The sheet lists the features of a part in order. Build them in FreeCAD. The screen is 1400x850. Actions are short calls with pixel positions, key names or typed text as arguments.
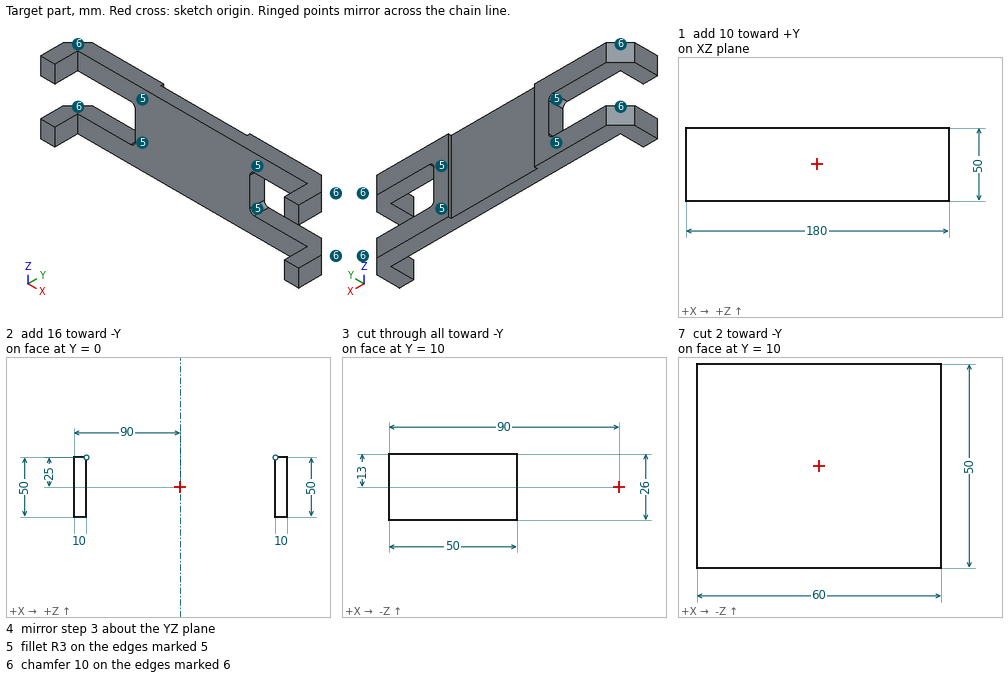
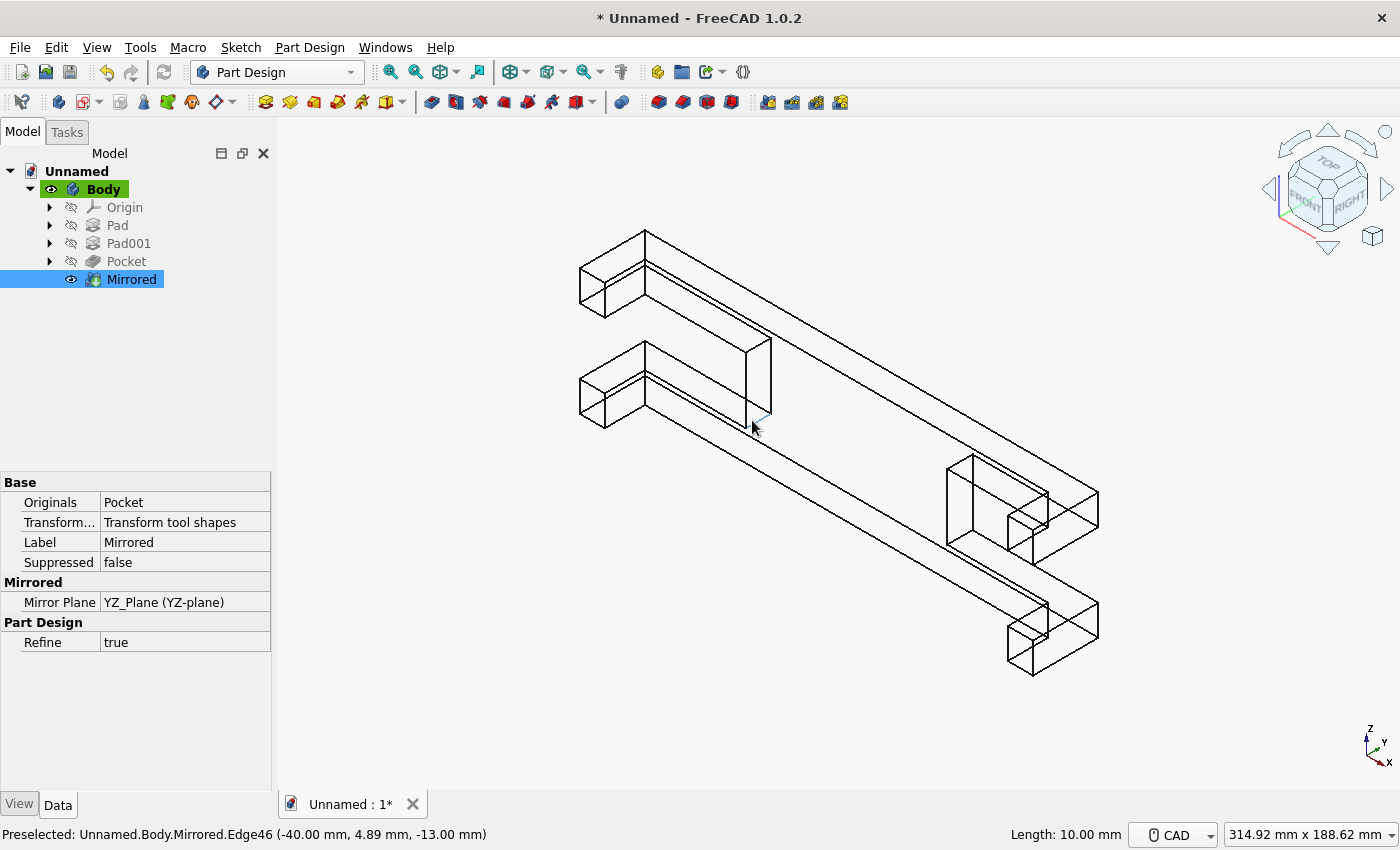
click(758, 344, ctrl)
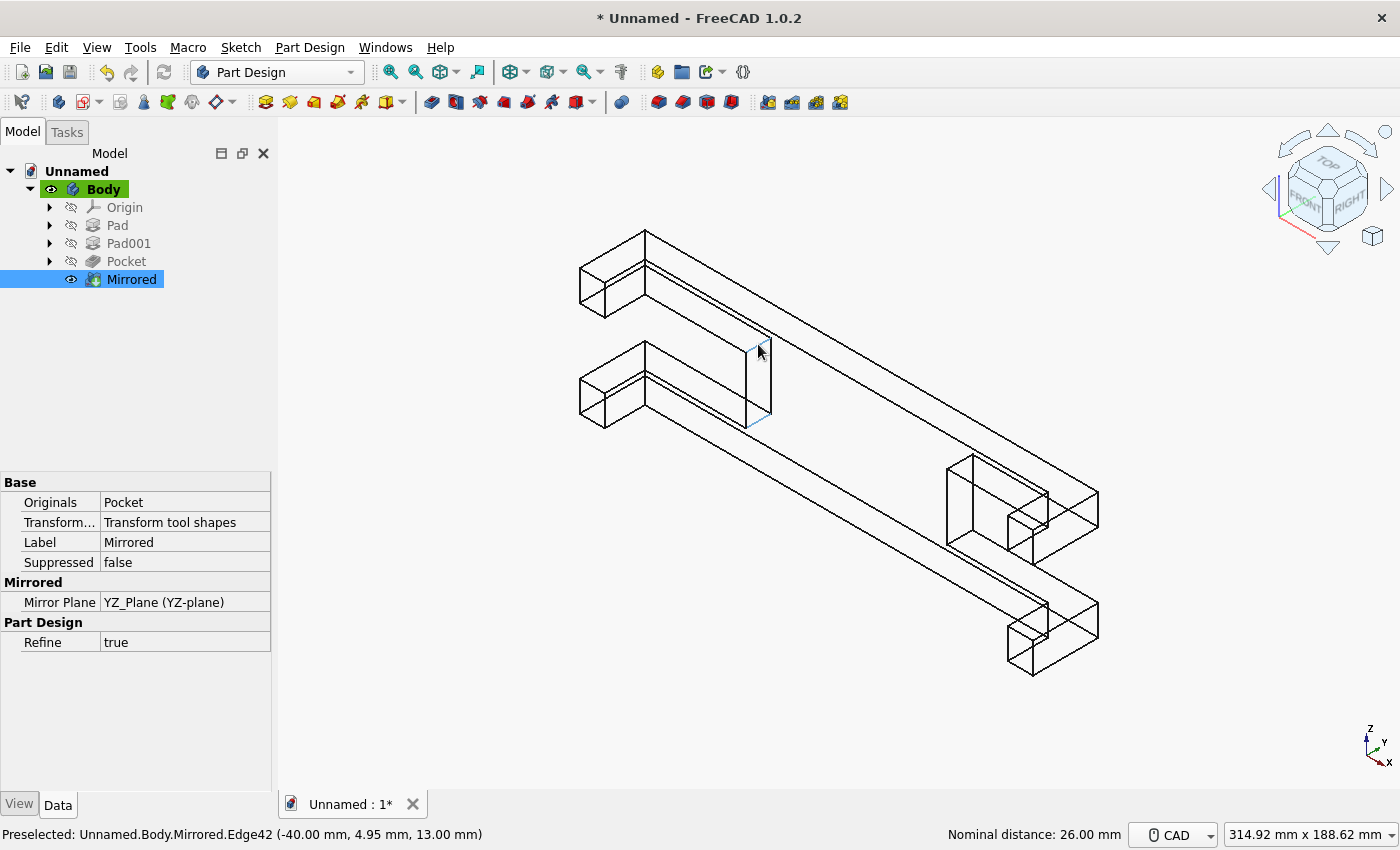
click(960, 461, ctrl)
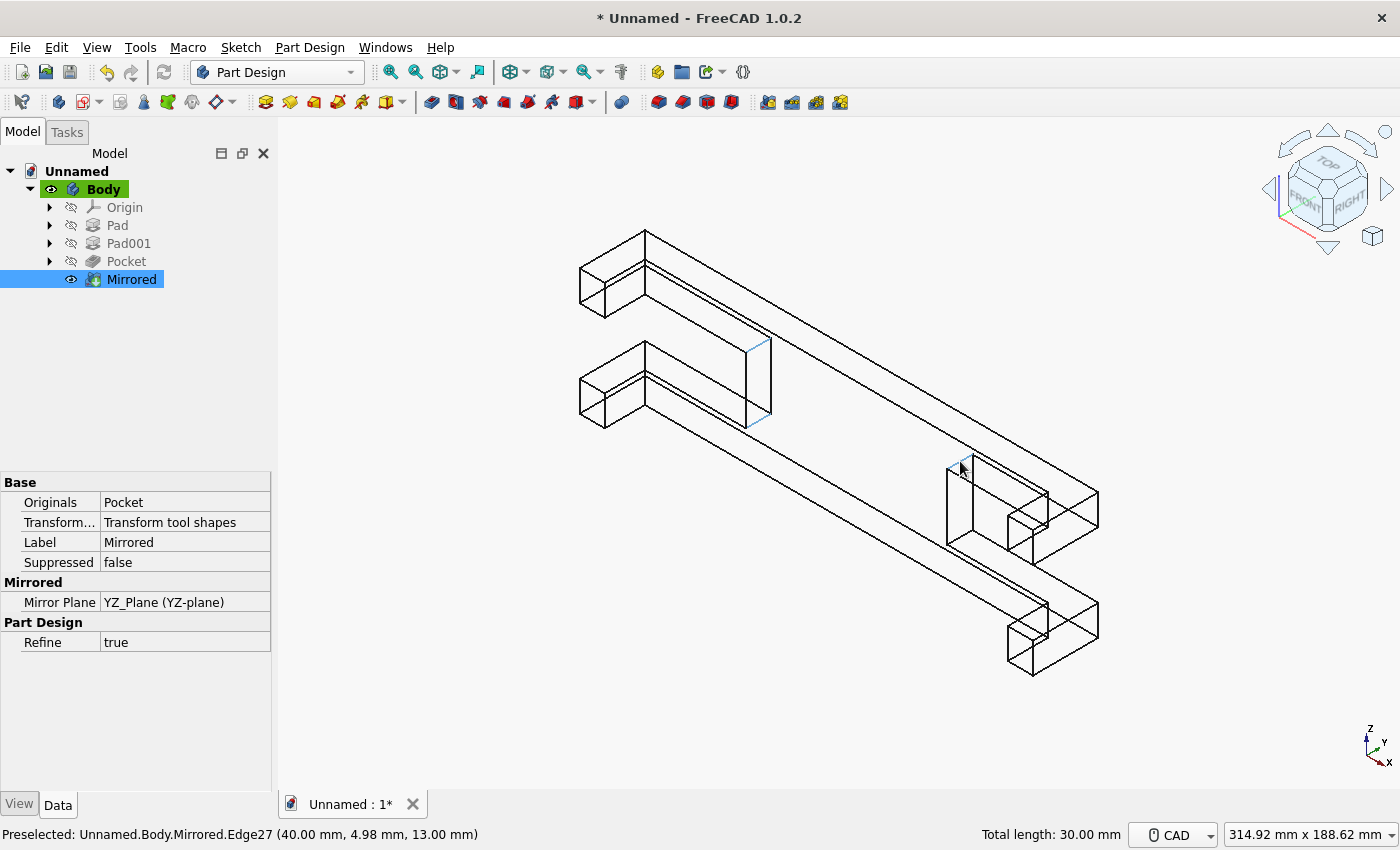
click(960, 536, ctrl)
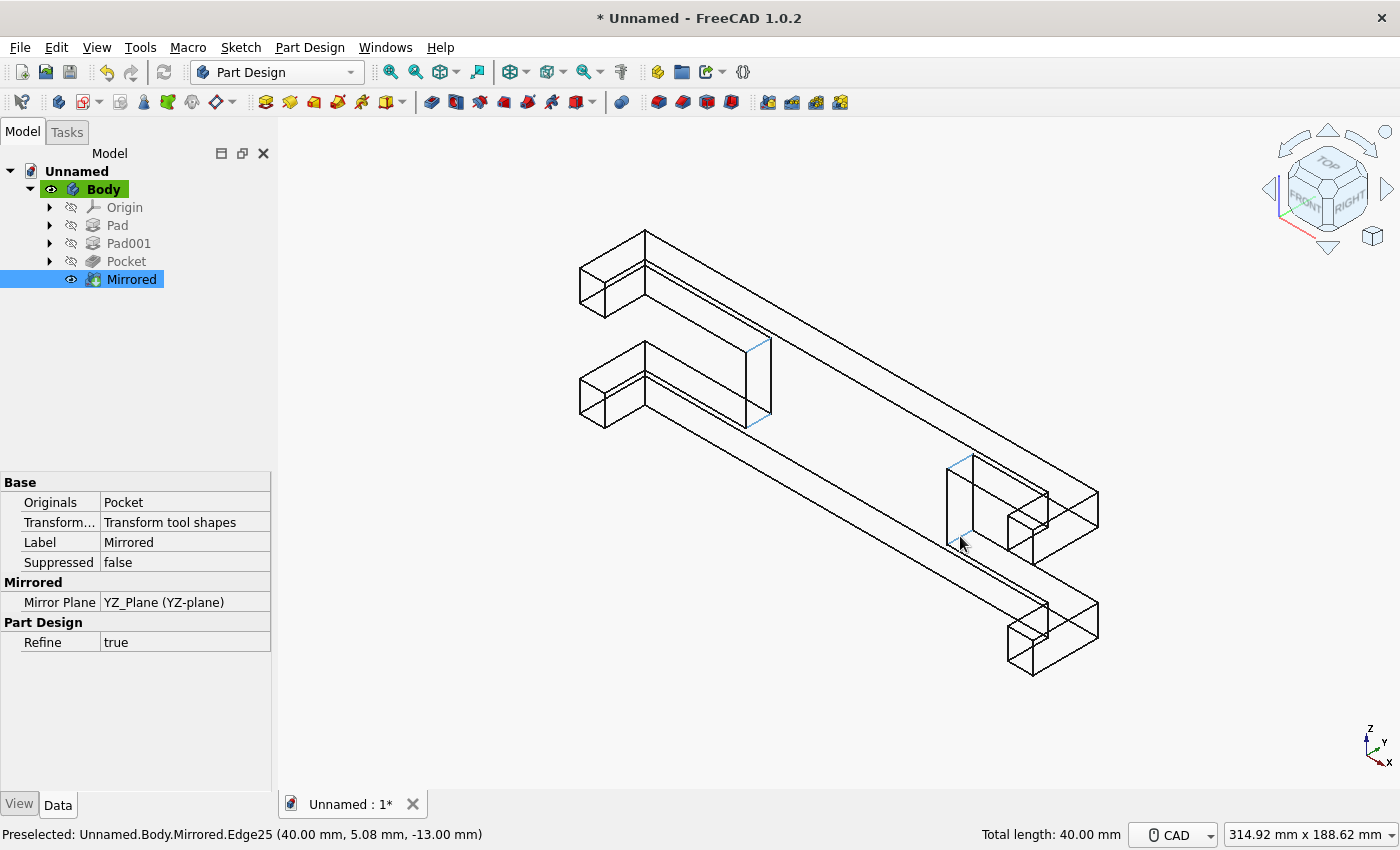
key(v)
key(1)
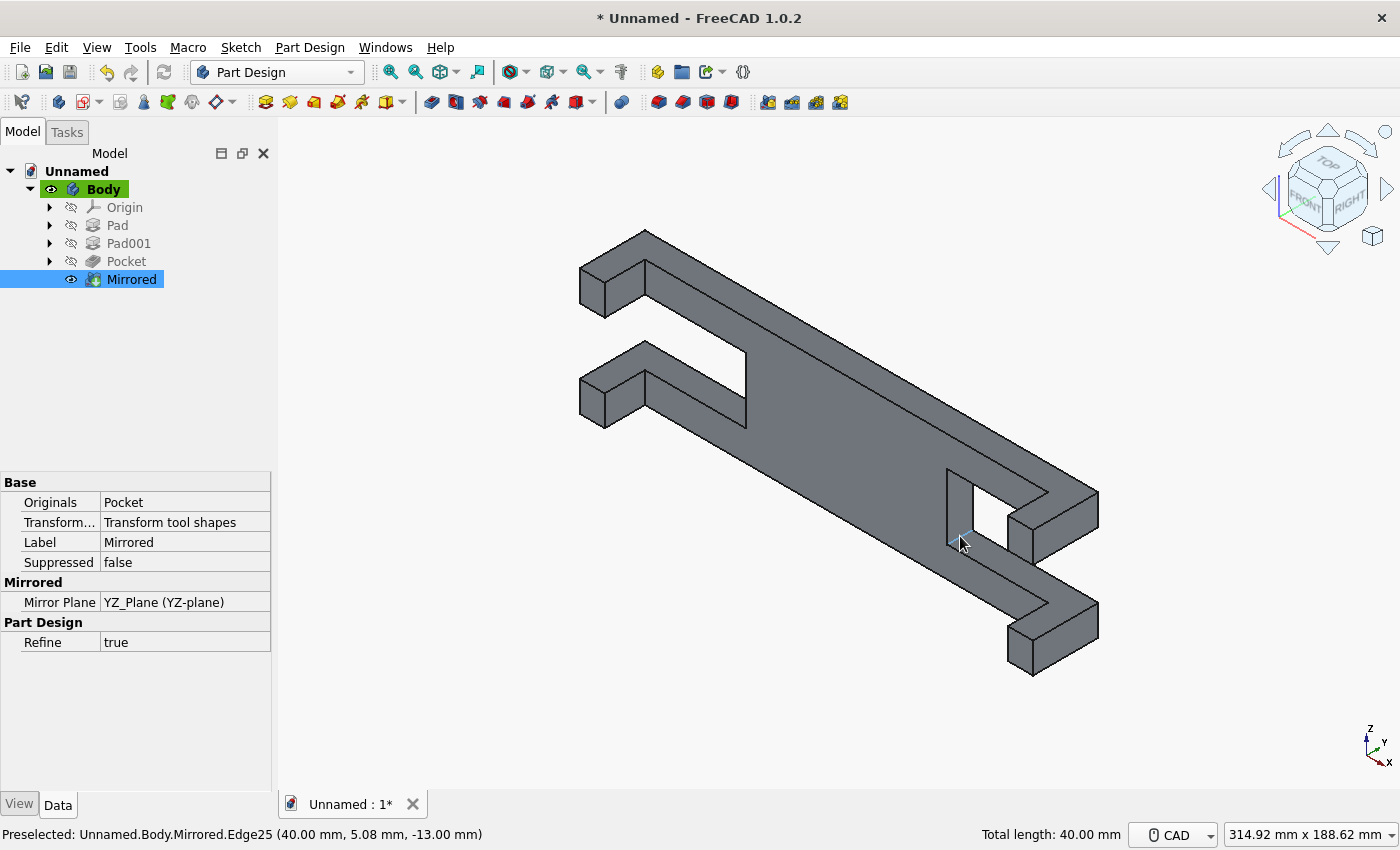
click(660, 102)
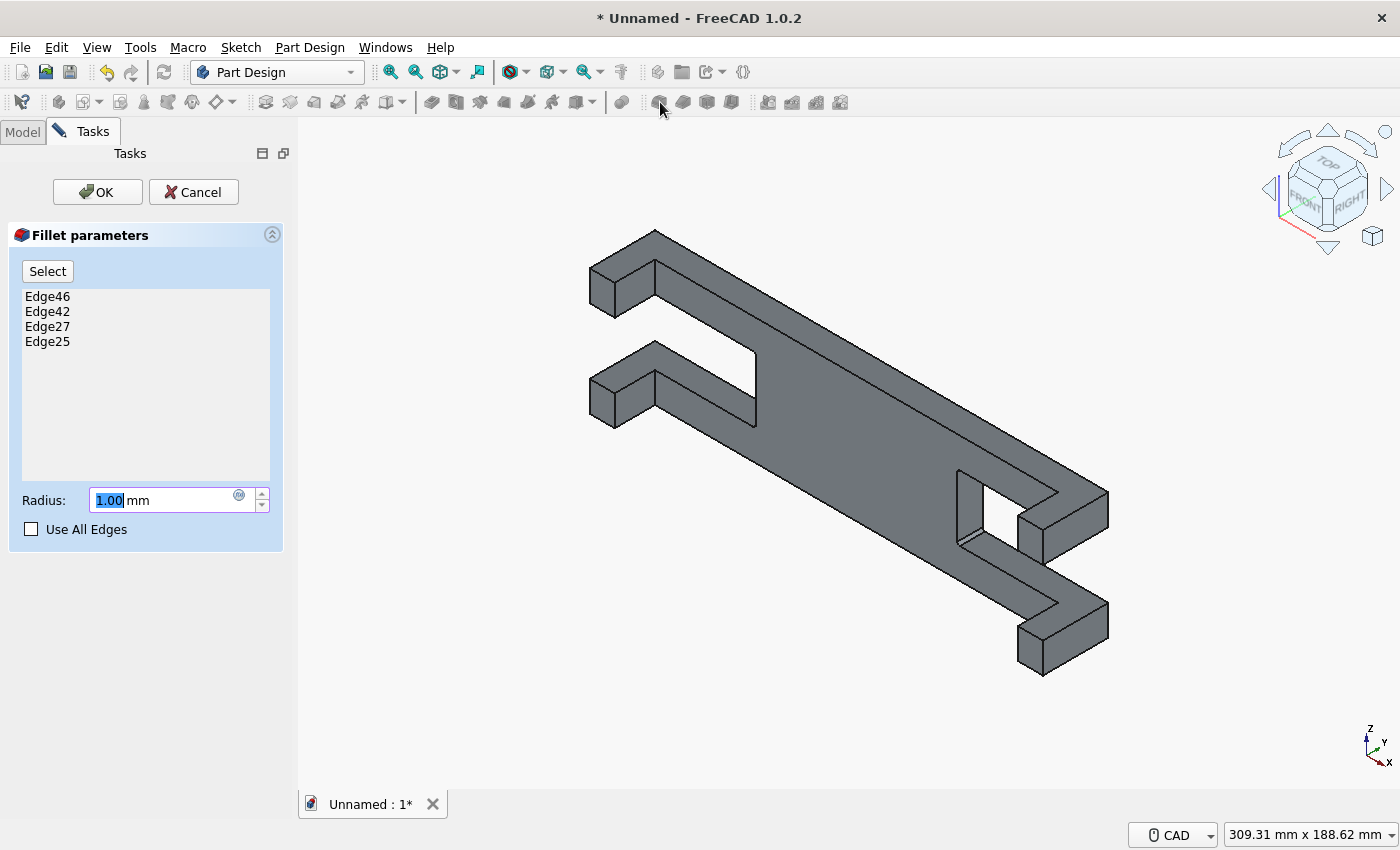
text(3)
key(Tab)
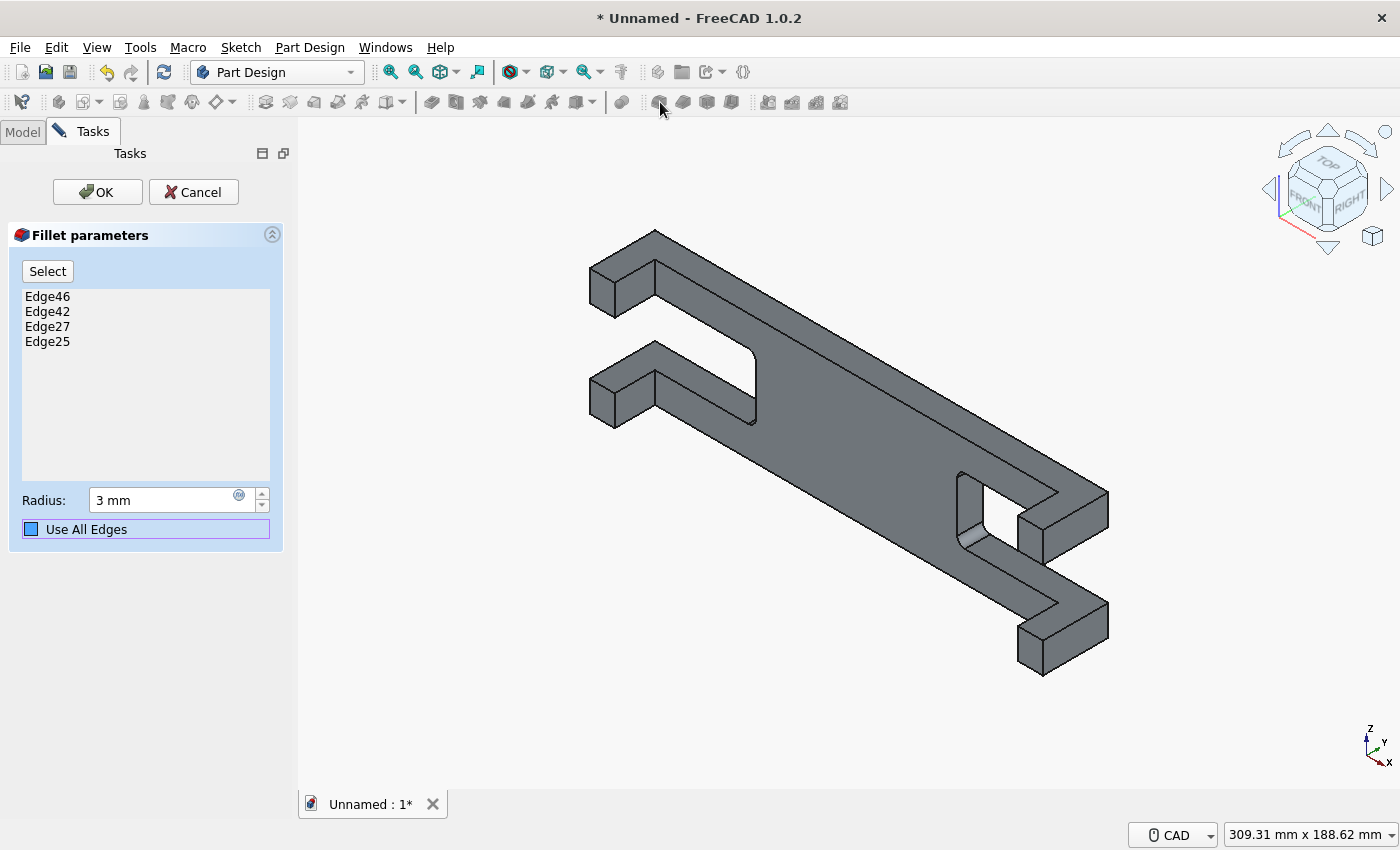
click(98, 192)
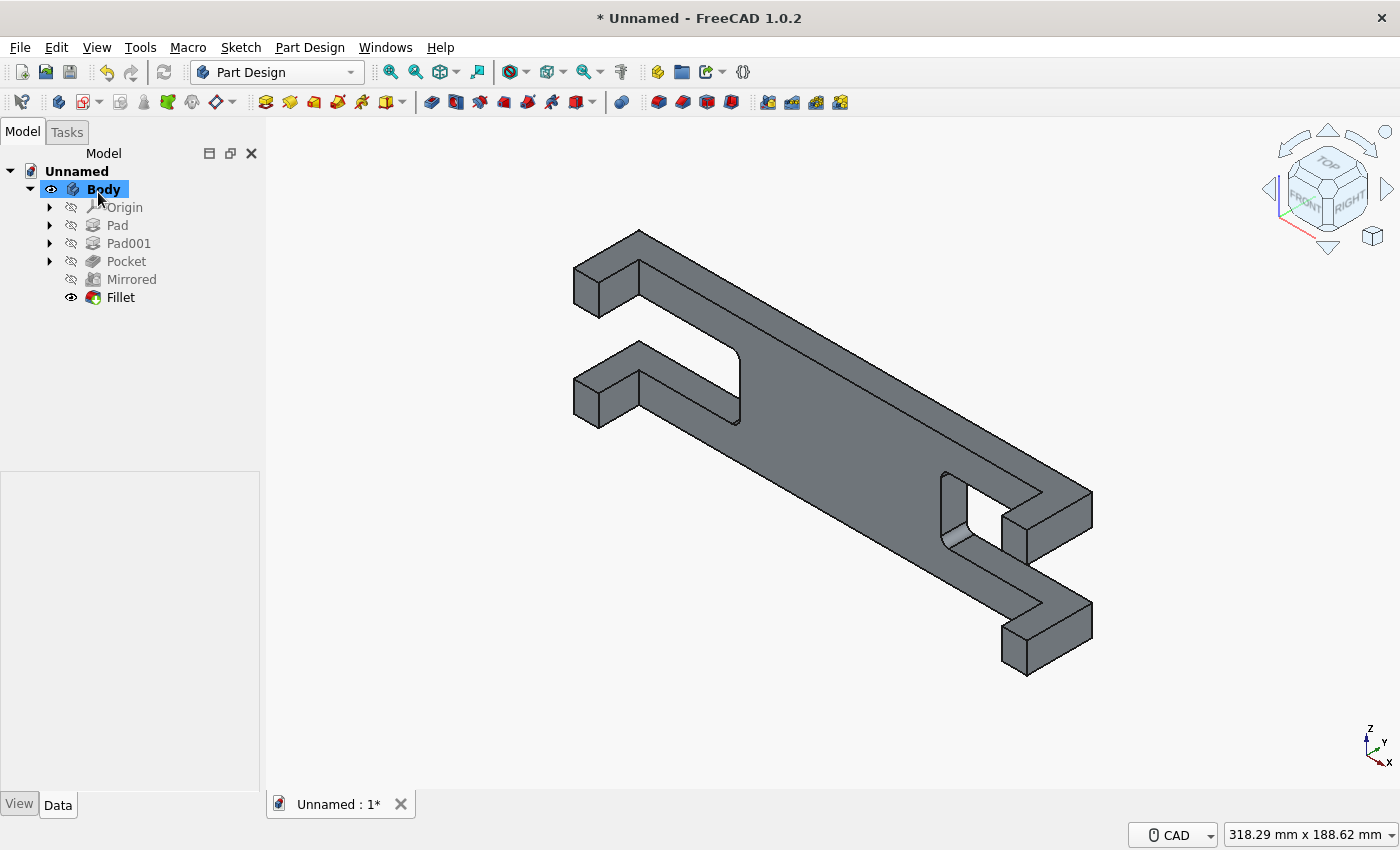
key(2)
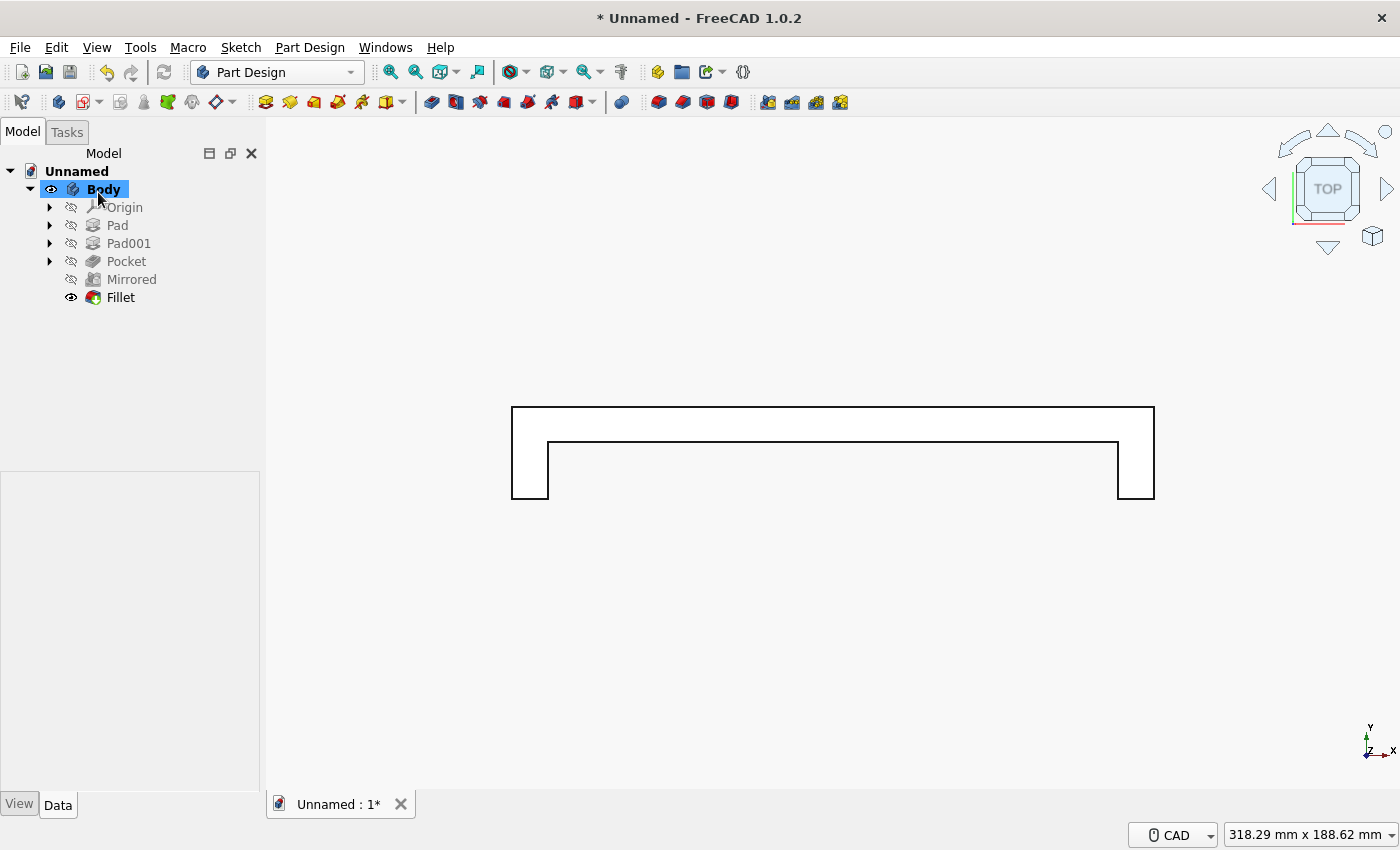
key(0)